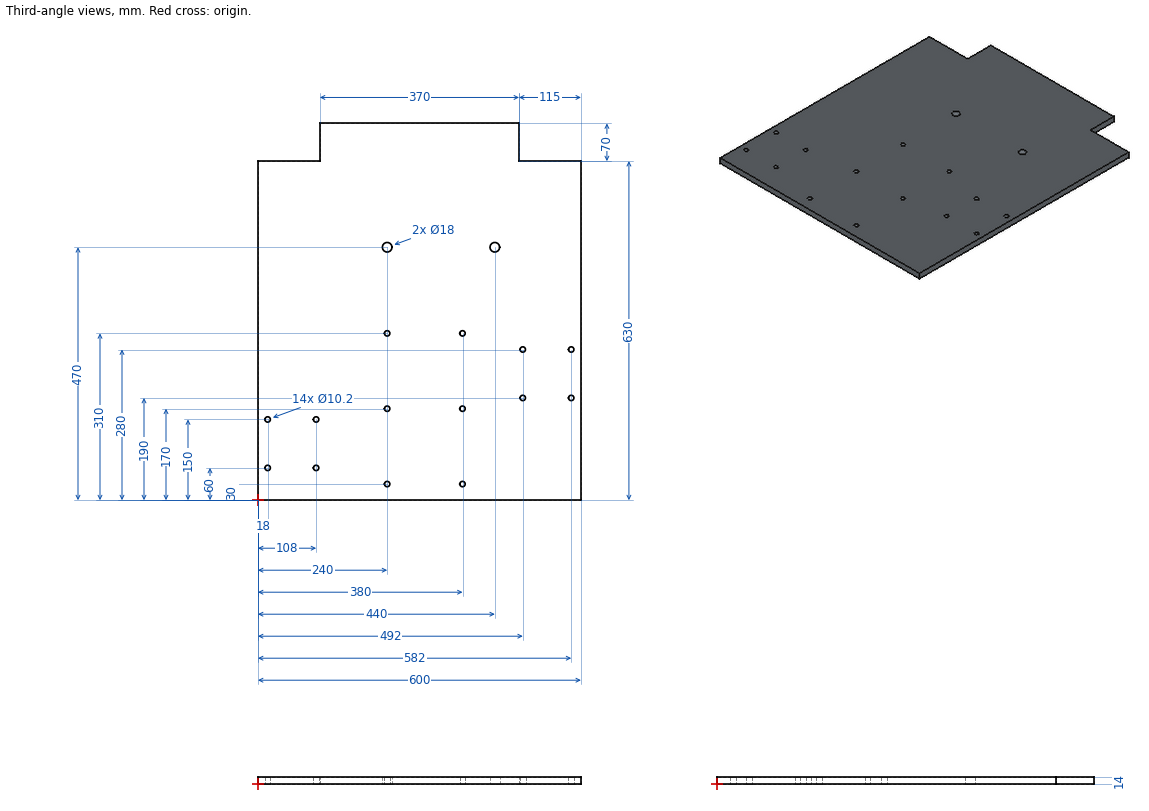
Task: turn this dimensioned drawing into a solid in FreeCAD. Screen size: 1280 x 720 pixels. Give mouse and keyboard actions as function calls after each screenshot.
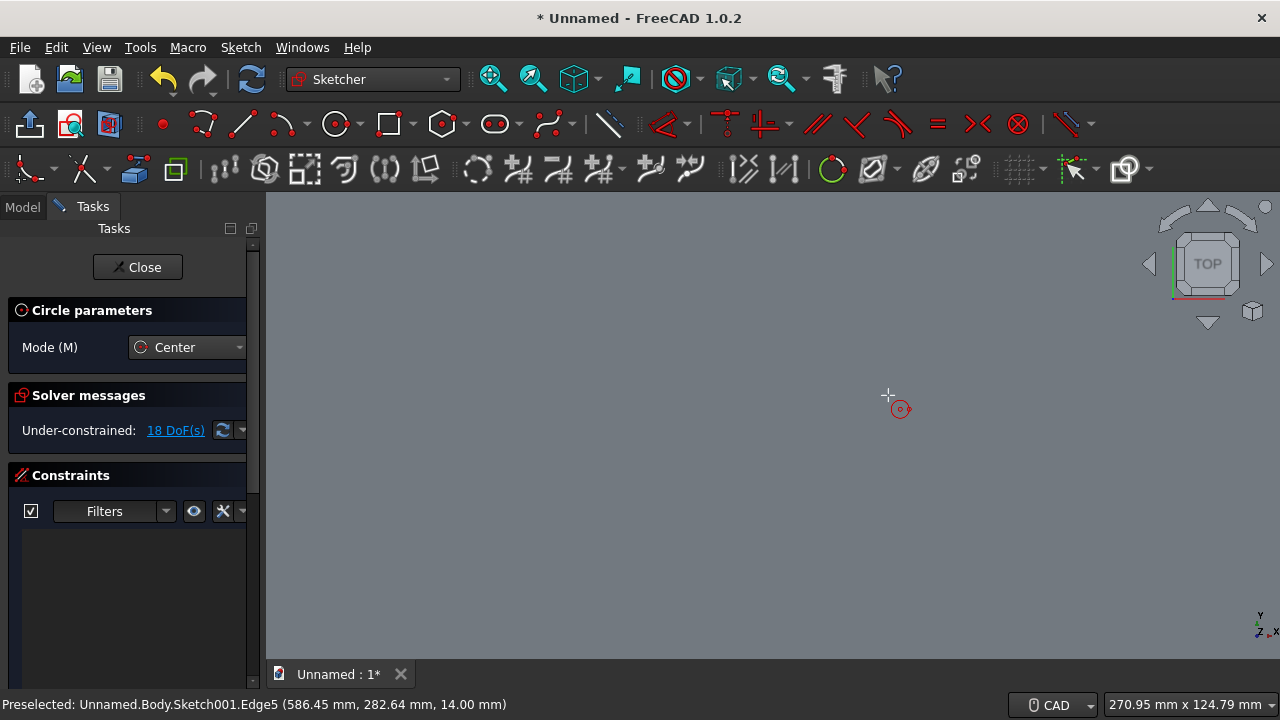
scroll(888, 396, down, 8)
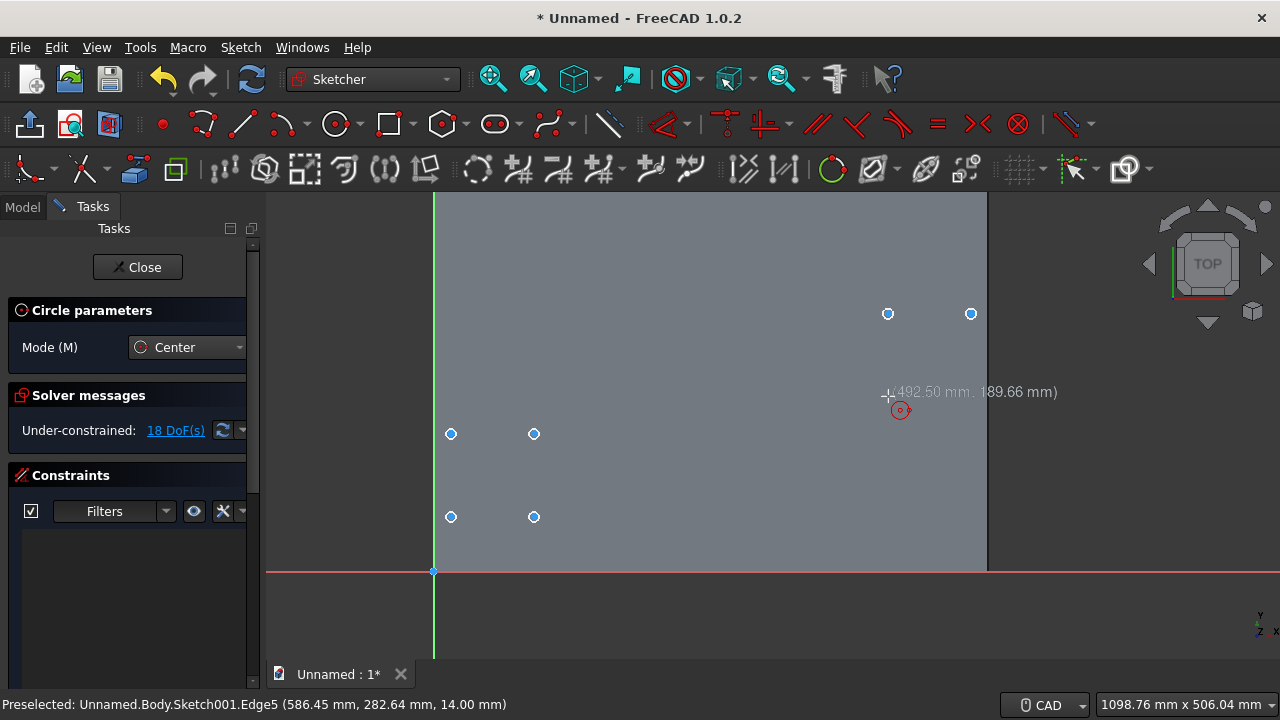
click(888, 396)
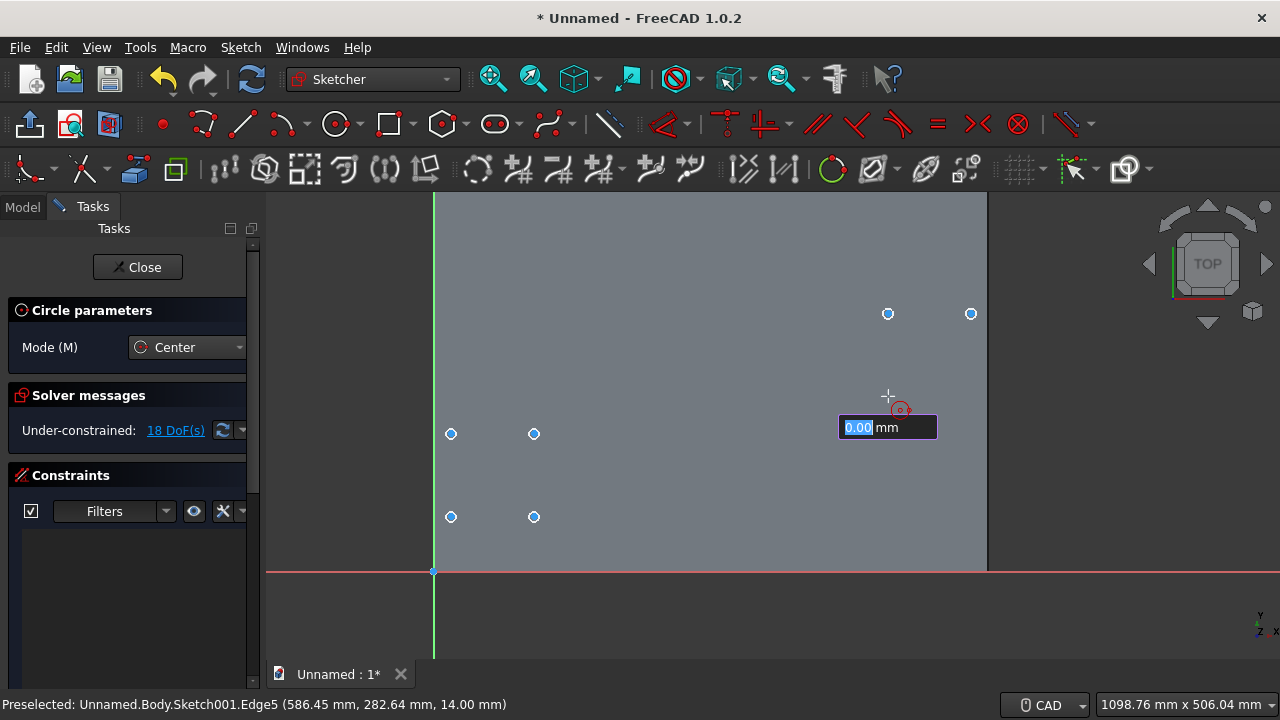
scroll(891, 393, up, 7)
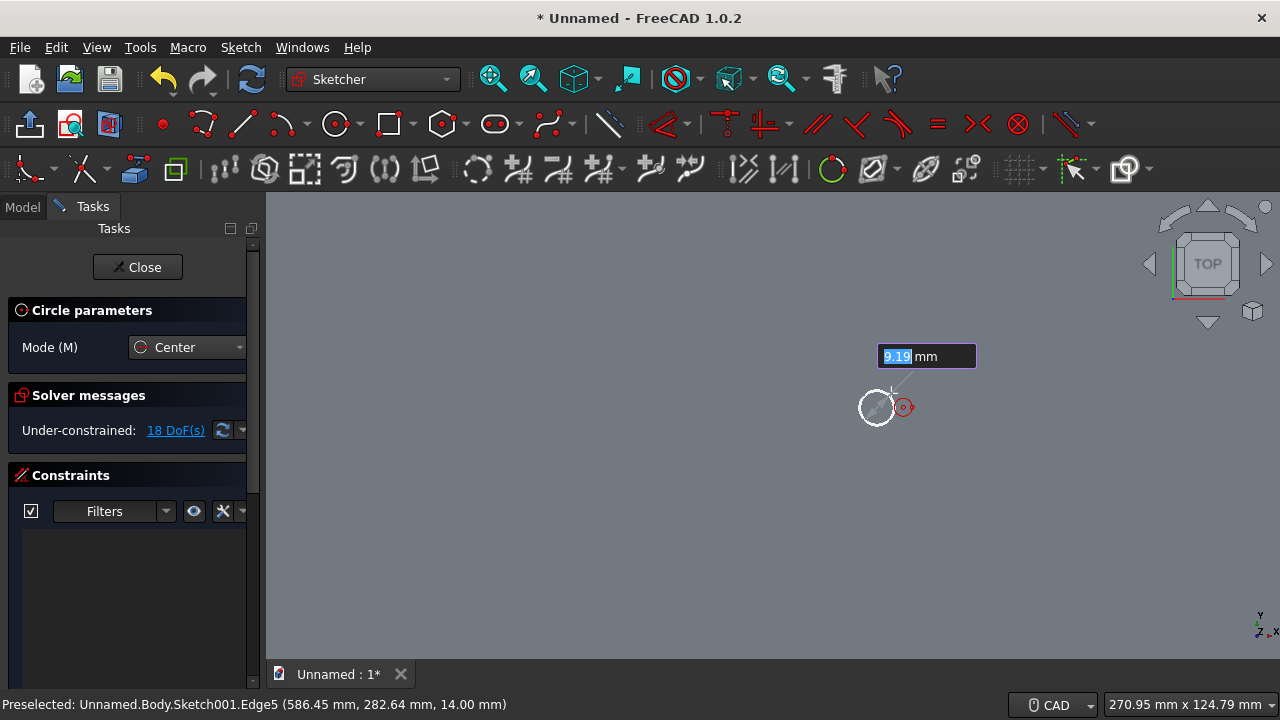
click(891, 391)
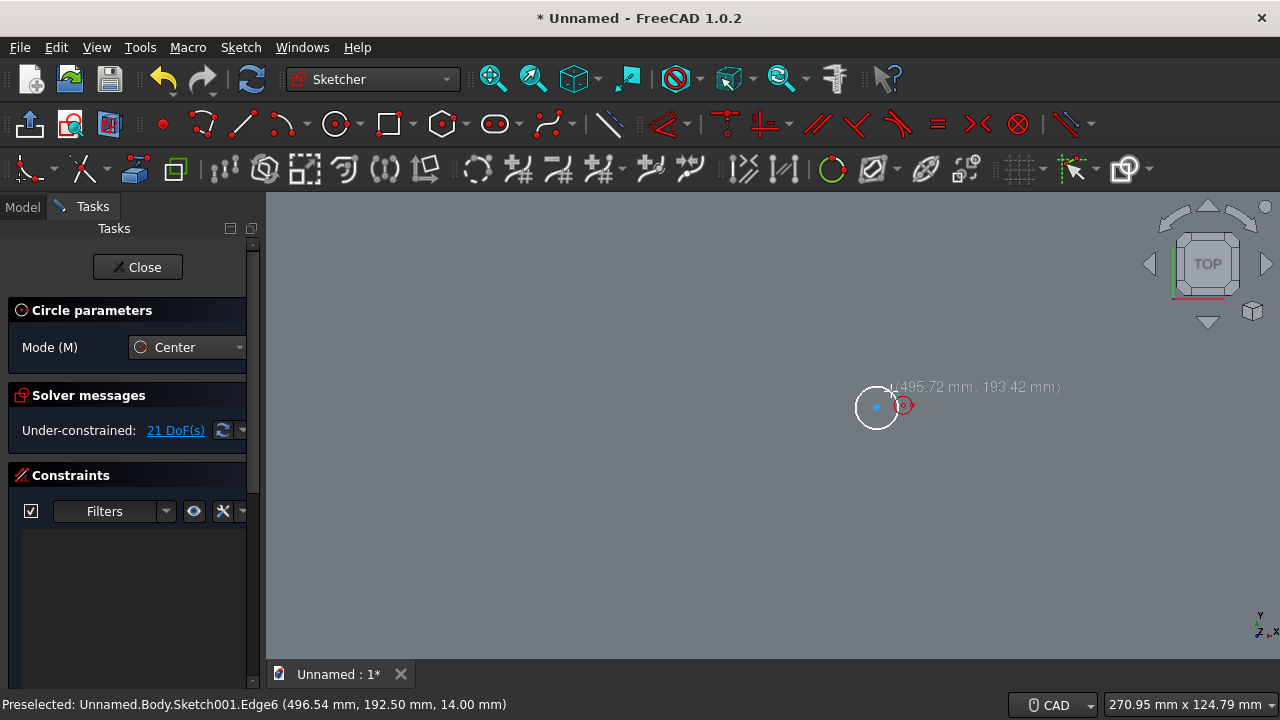
scroll(891, 393, down, 7)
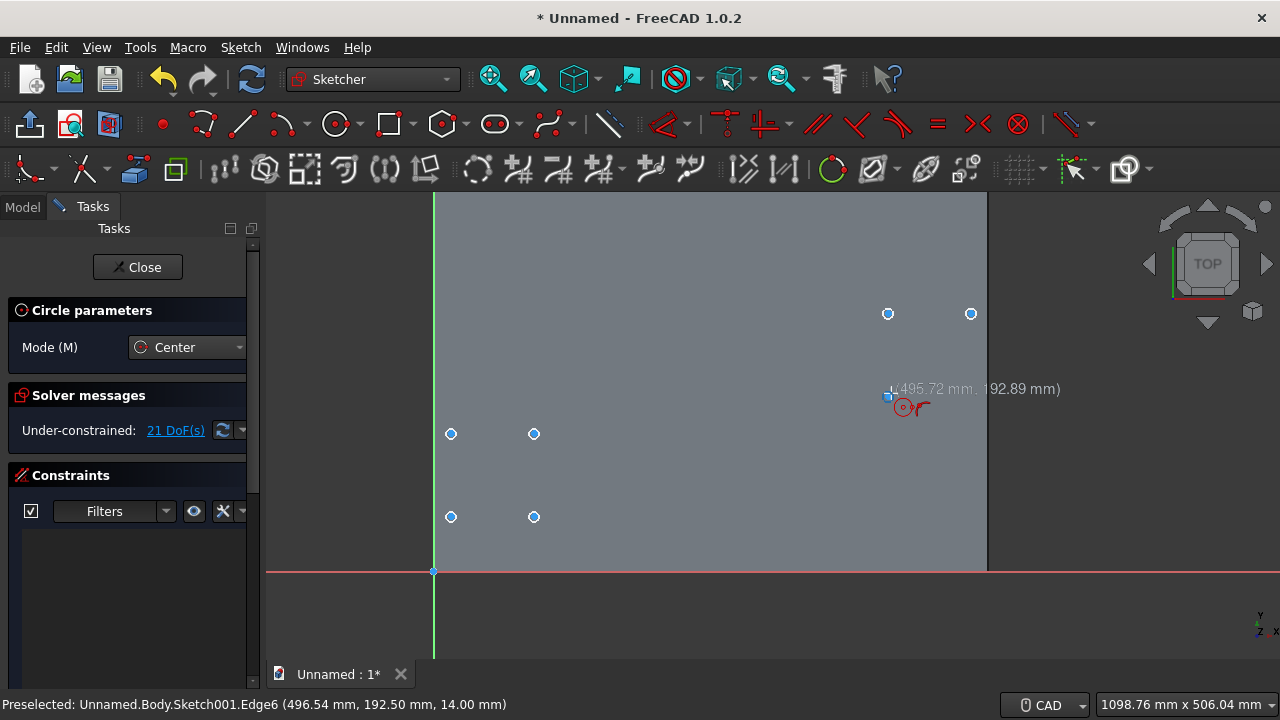
scroll(971, 396, up, 8)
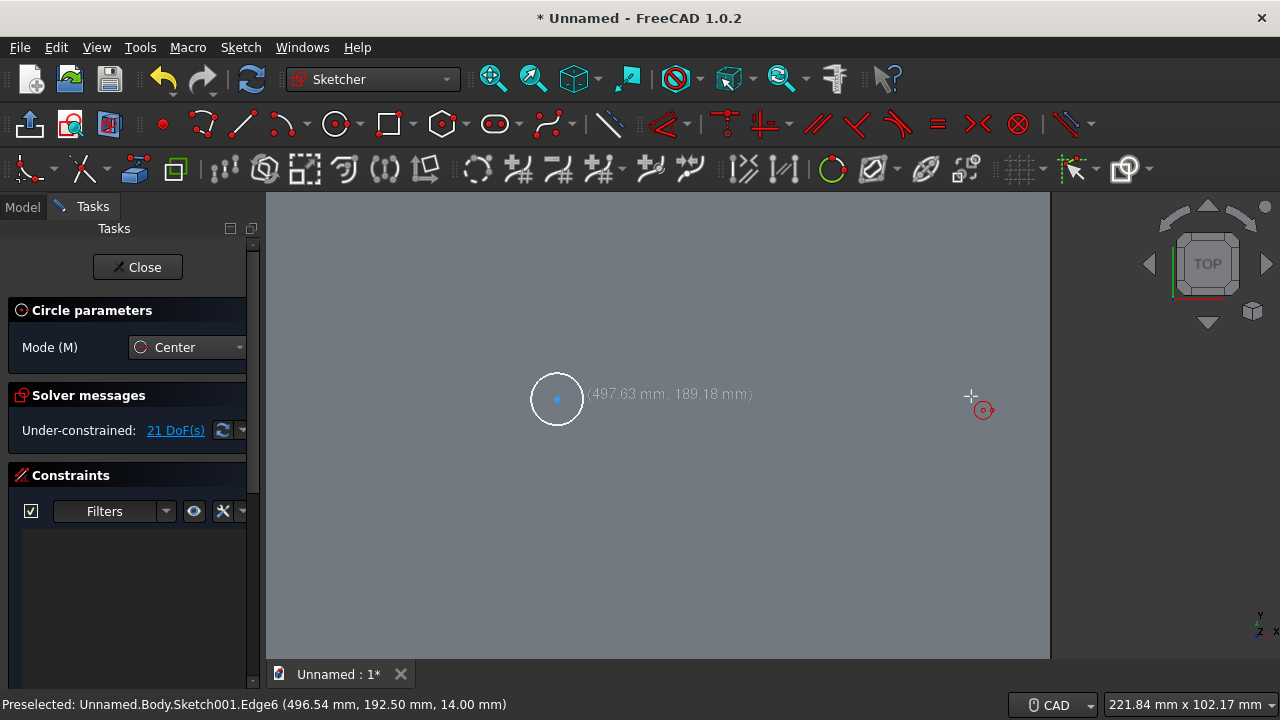
scroll(971, 396, down, 8)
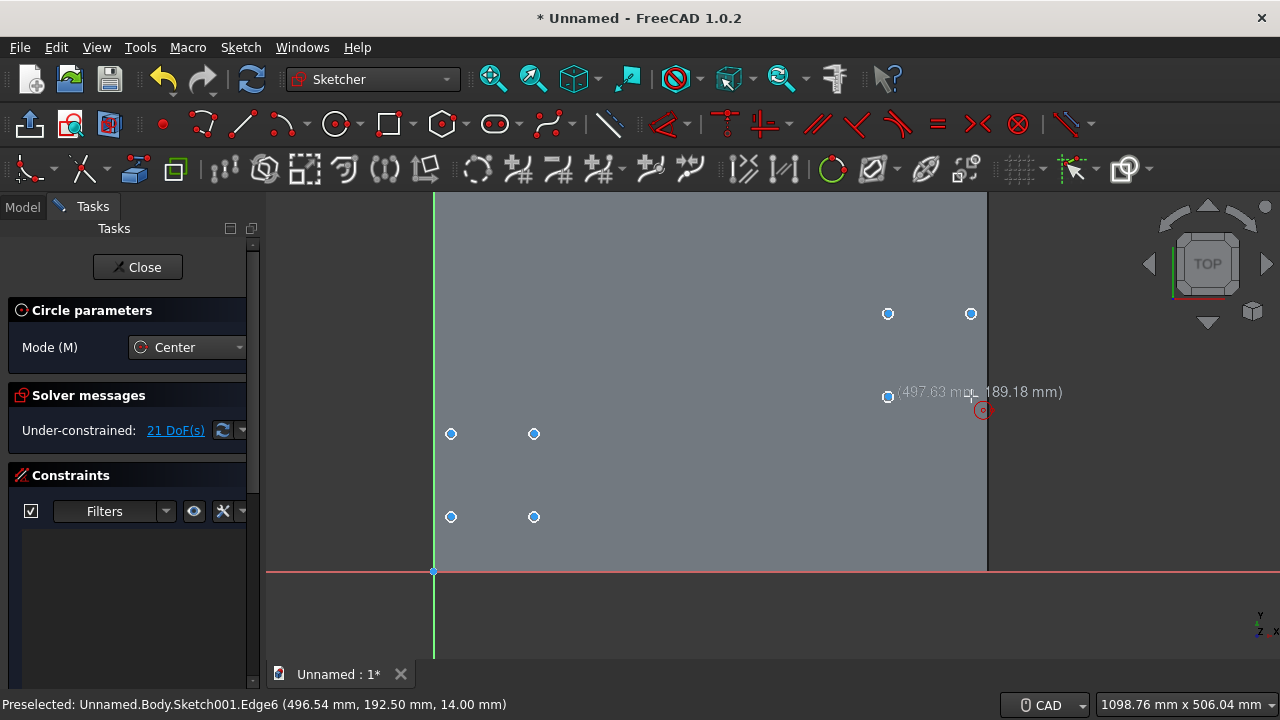
click(971, 396)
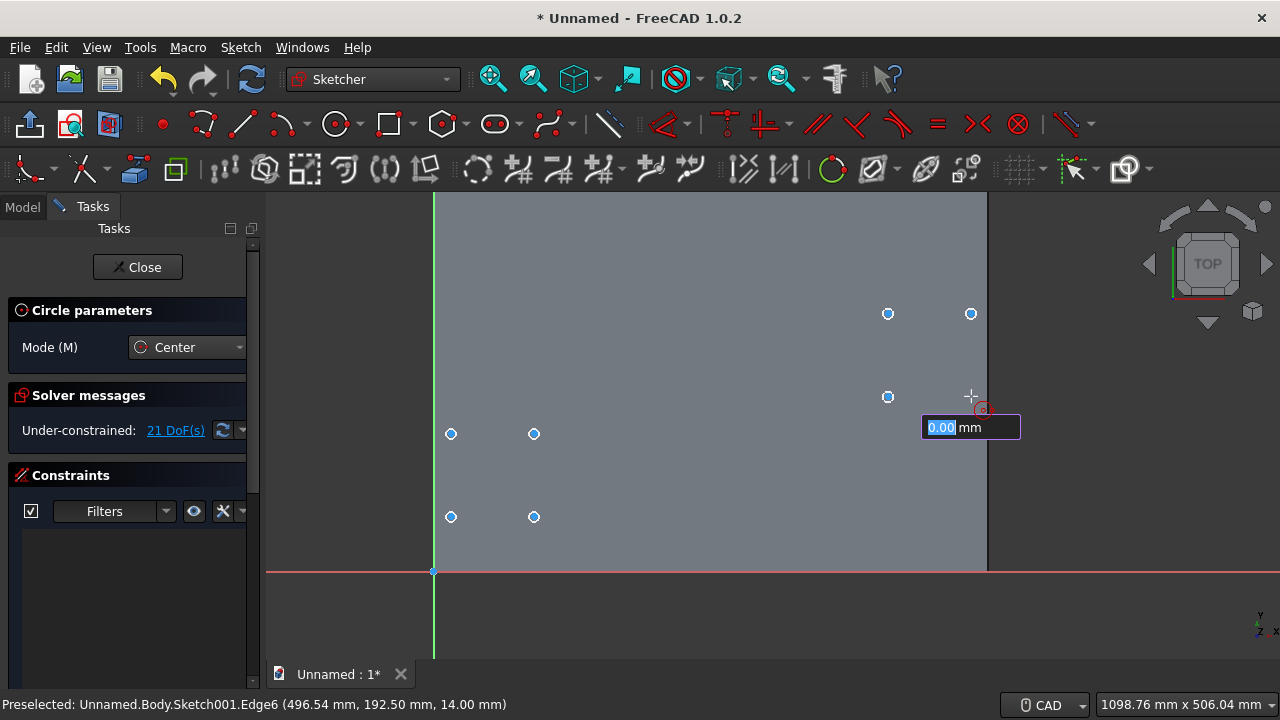
scroll(974, 393, up, 7)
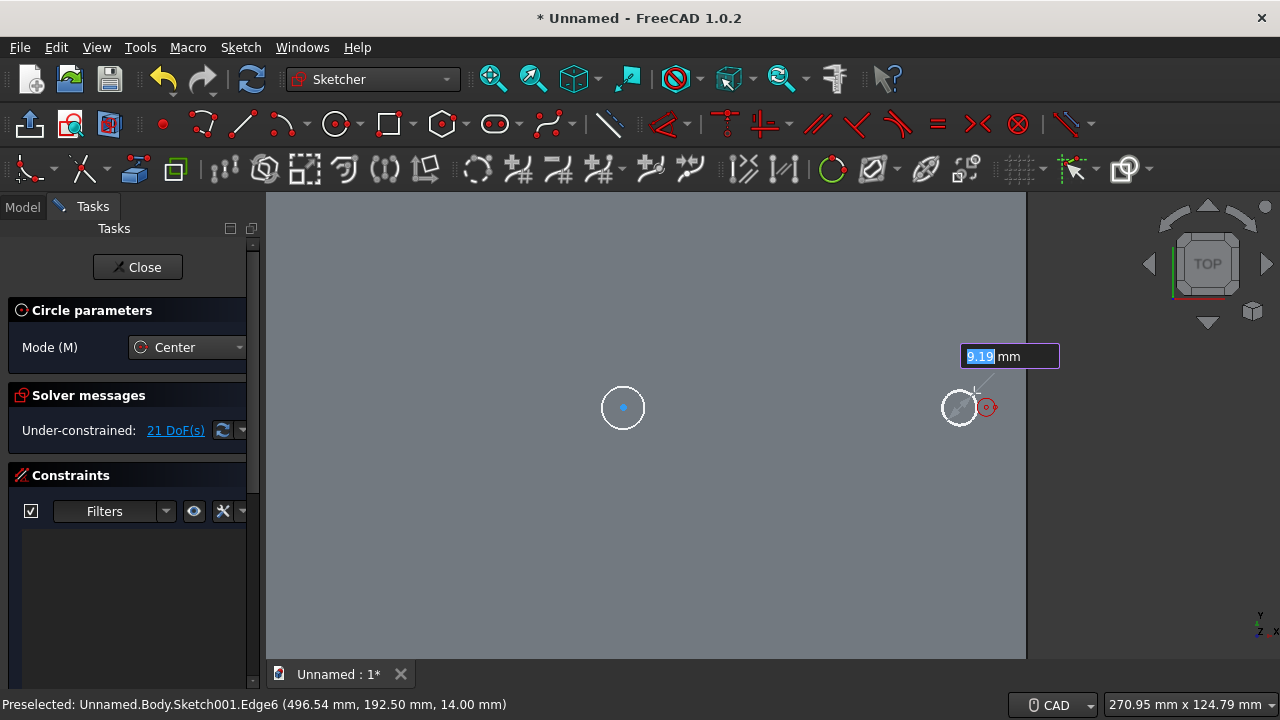
click(974, 391)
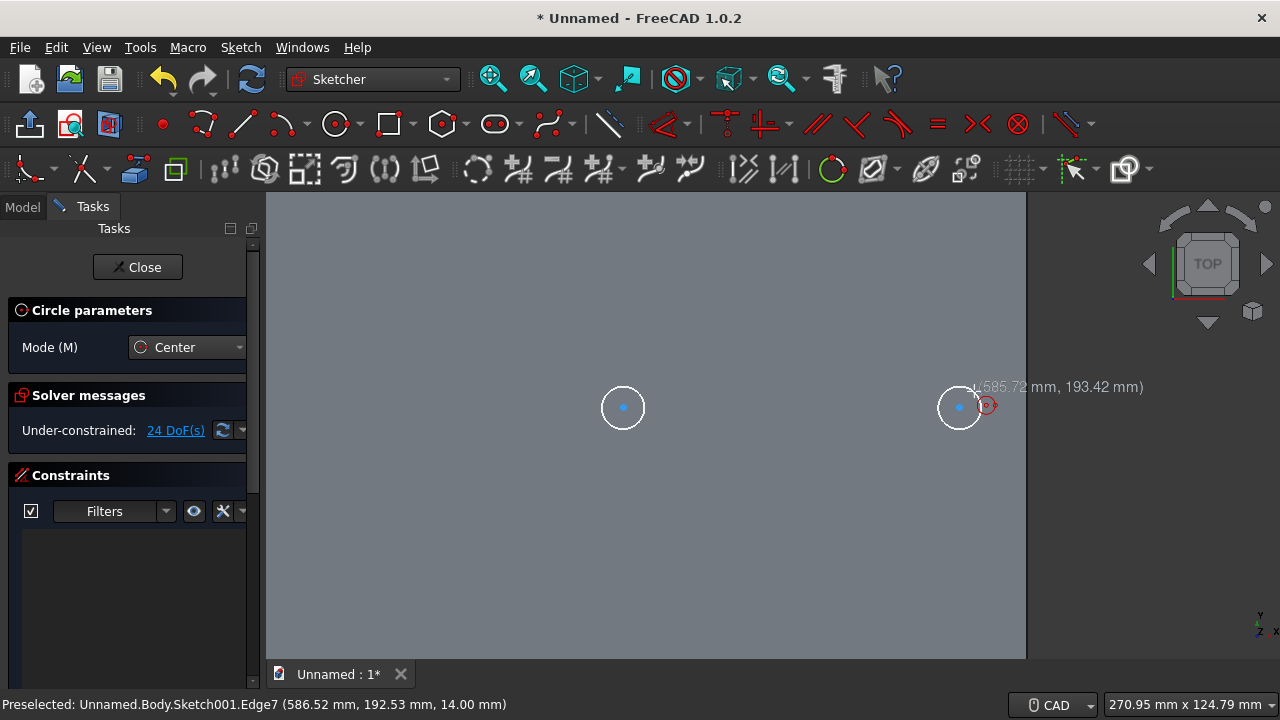
scroll(974, 393, down, 7)